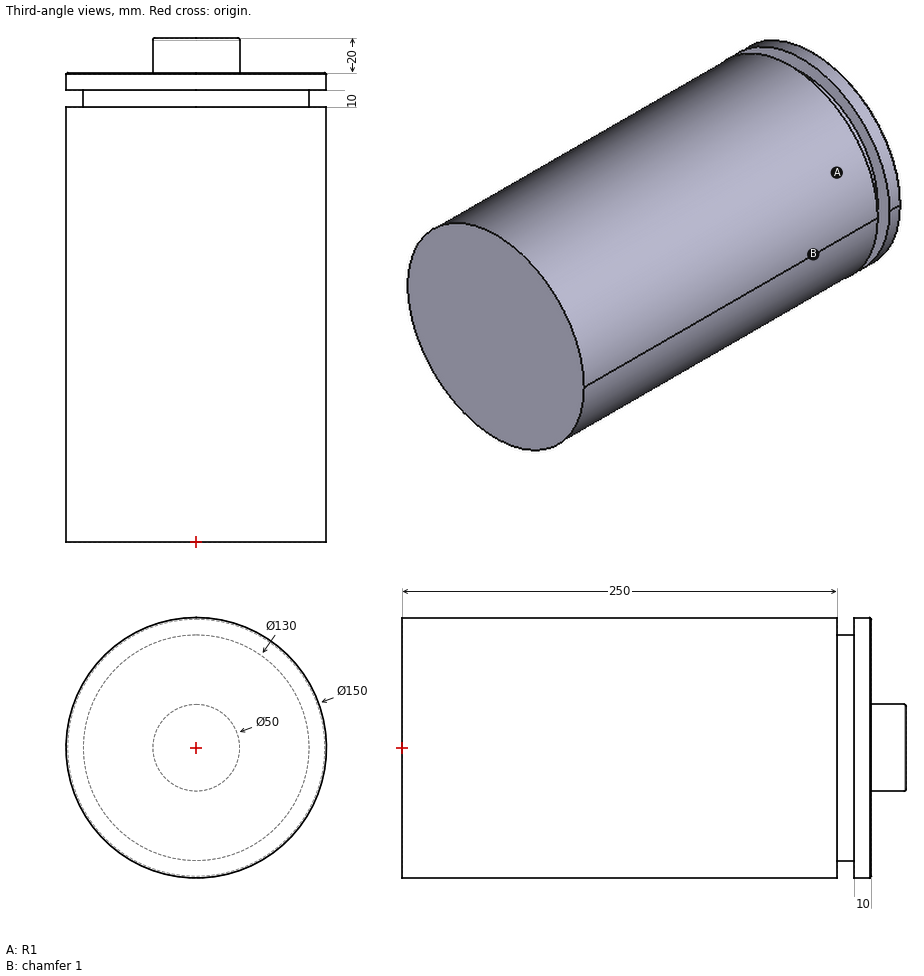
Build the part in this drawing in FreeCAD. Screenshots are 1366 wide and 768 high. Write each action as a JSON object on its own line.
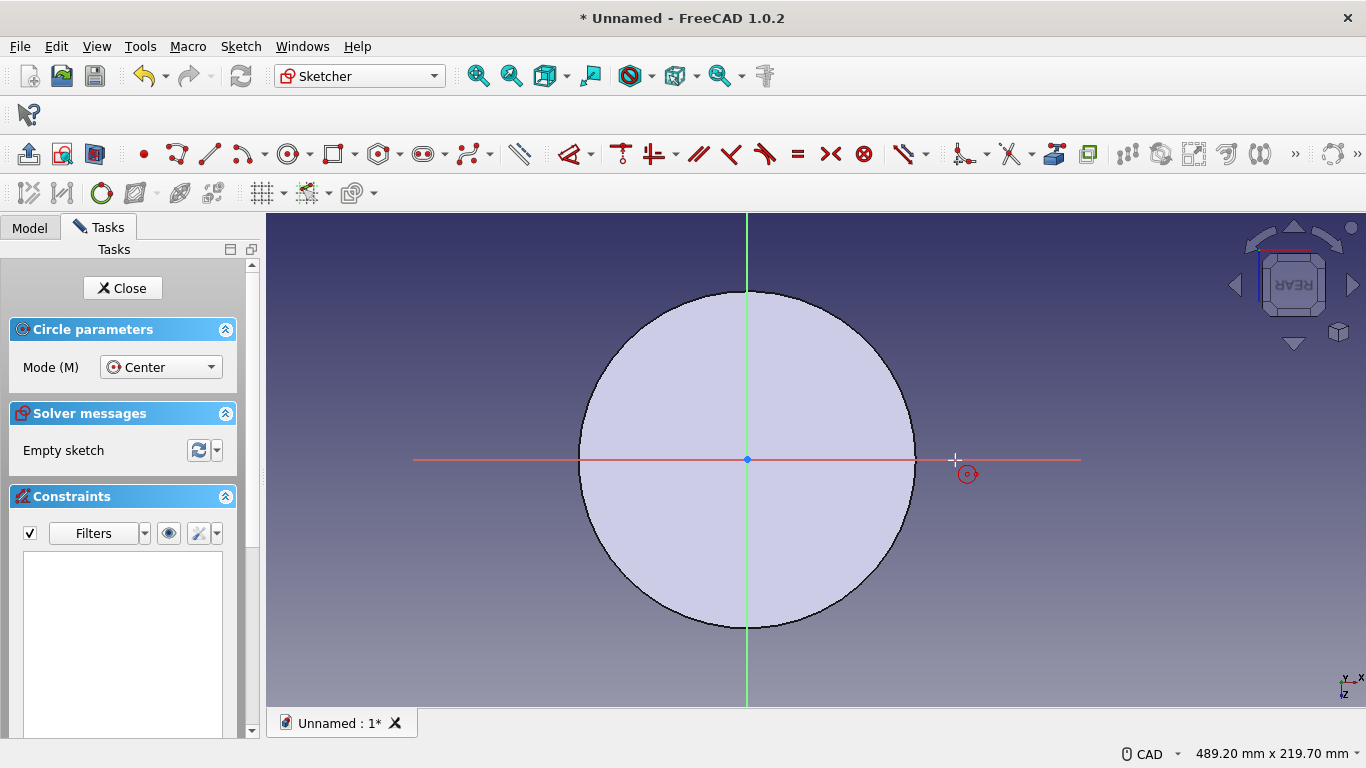
{"action": "left_click", "coordinate": [747, 460]}
{"action": "mouse_move", "coordinate": [850, 356]}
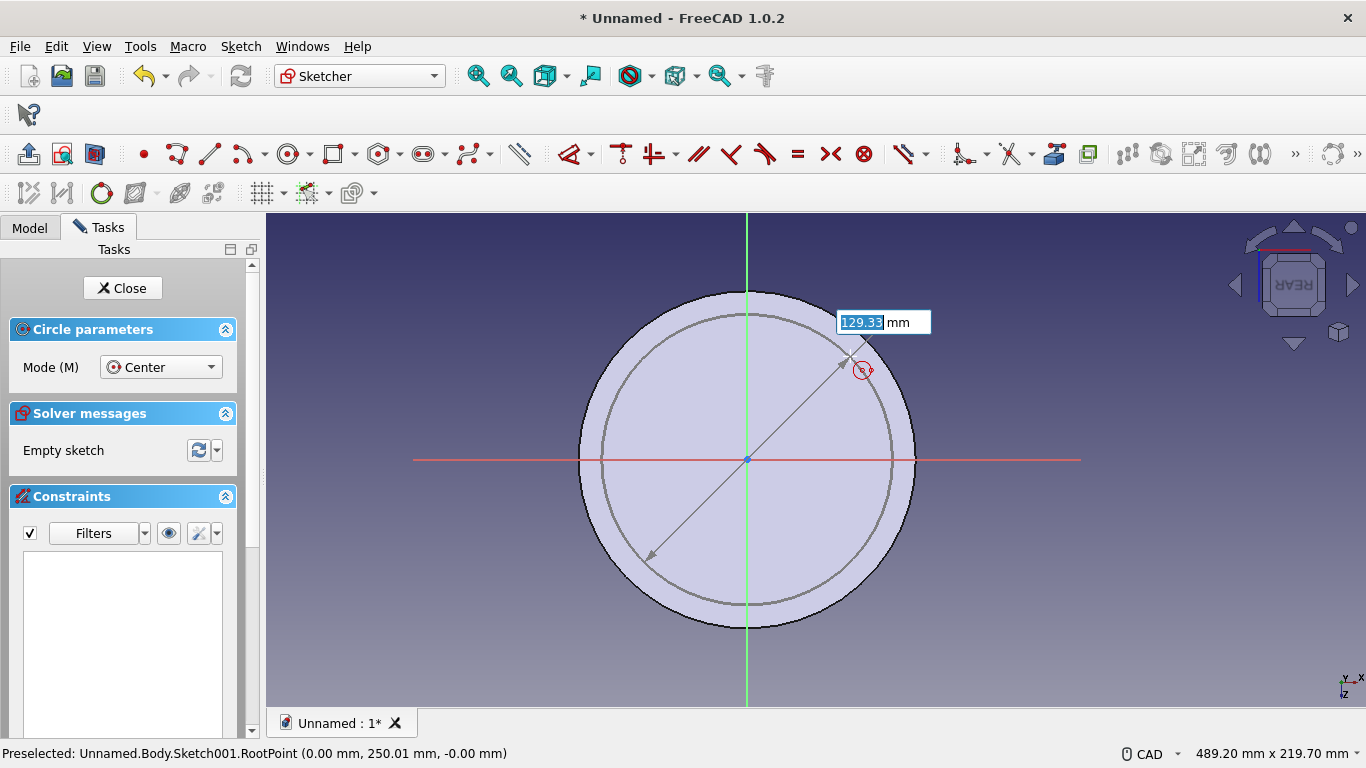
{"action": "type", "text": "130"}
{"action": "key", "text": "Return"}
{"action": "key", "text": "Escape"}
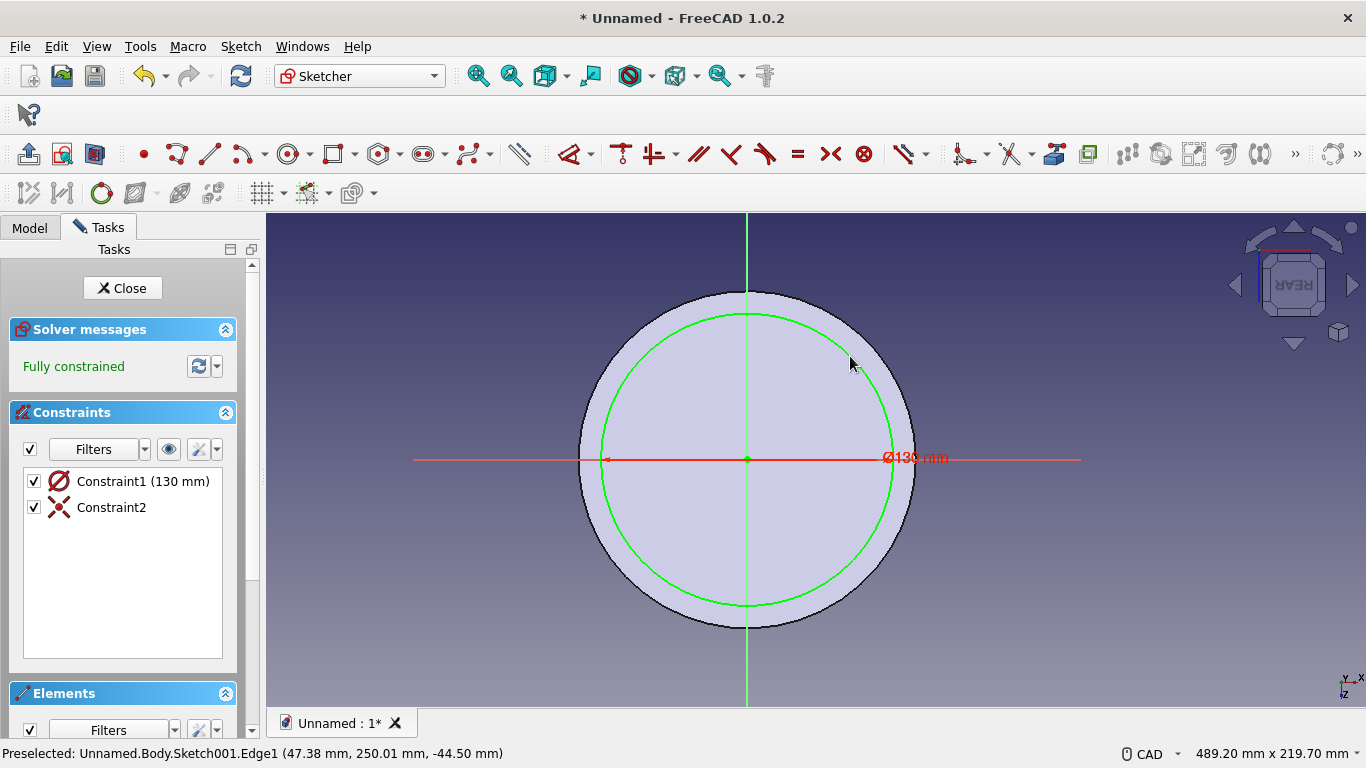
{"action": "left_click", "coordinate": [123, 288]}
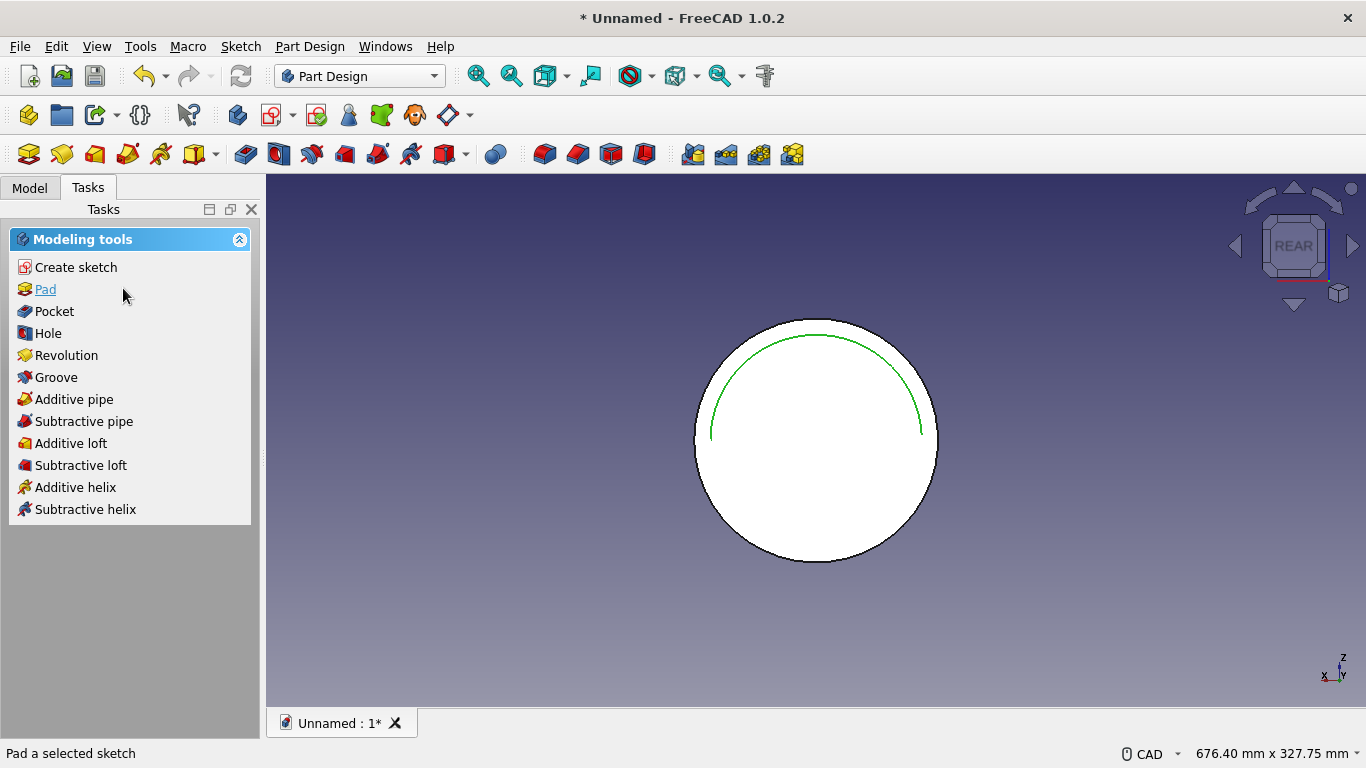
{"action": "left_click", "coordinate": [29, 154]}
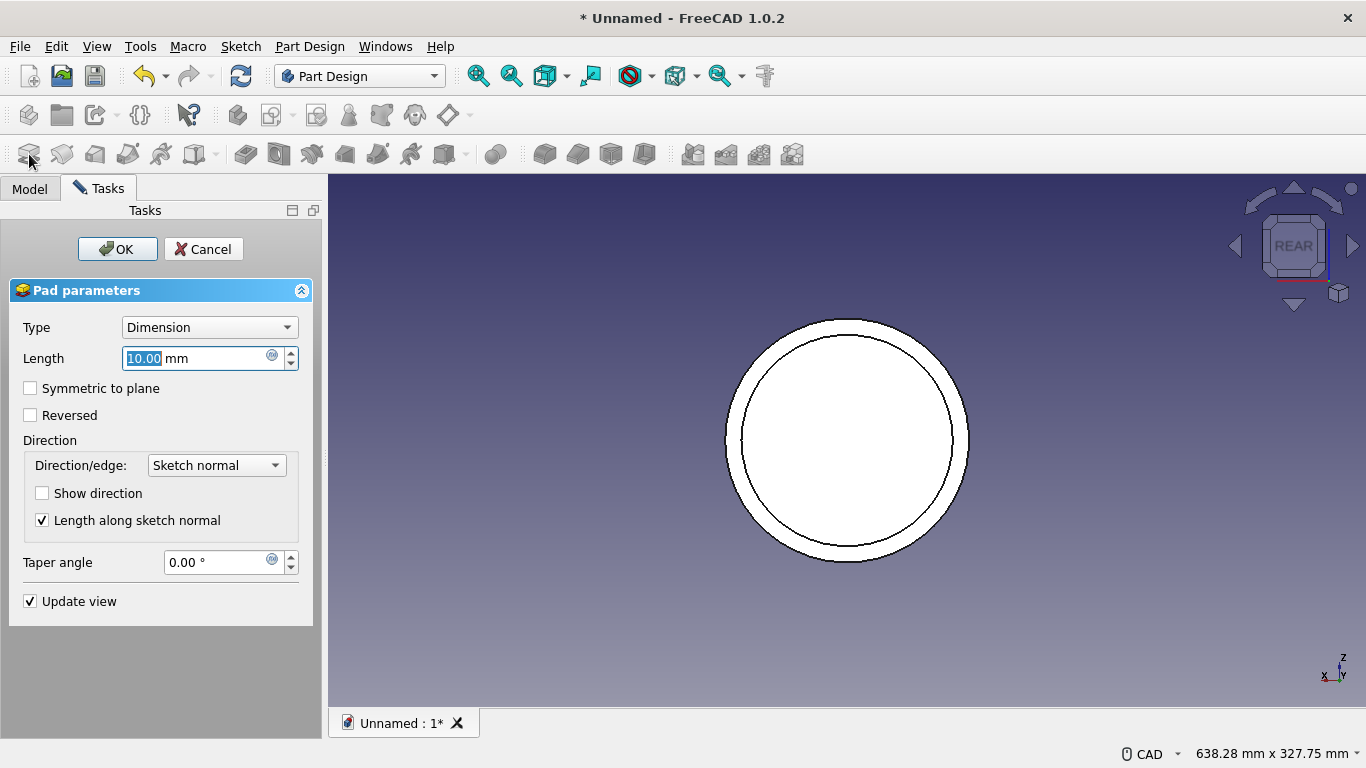
{"action": "type", "text": "10"}
{"action": "key", "text": "Tab"}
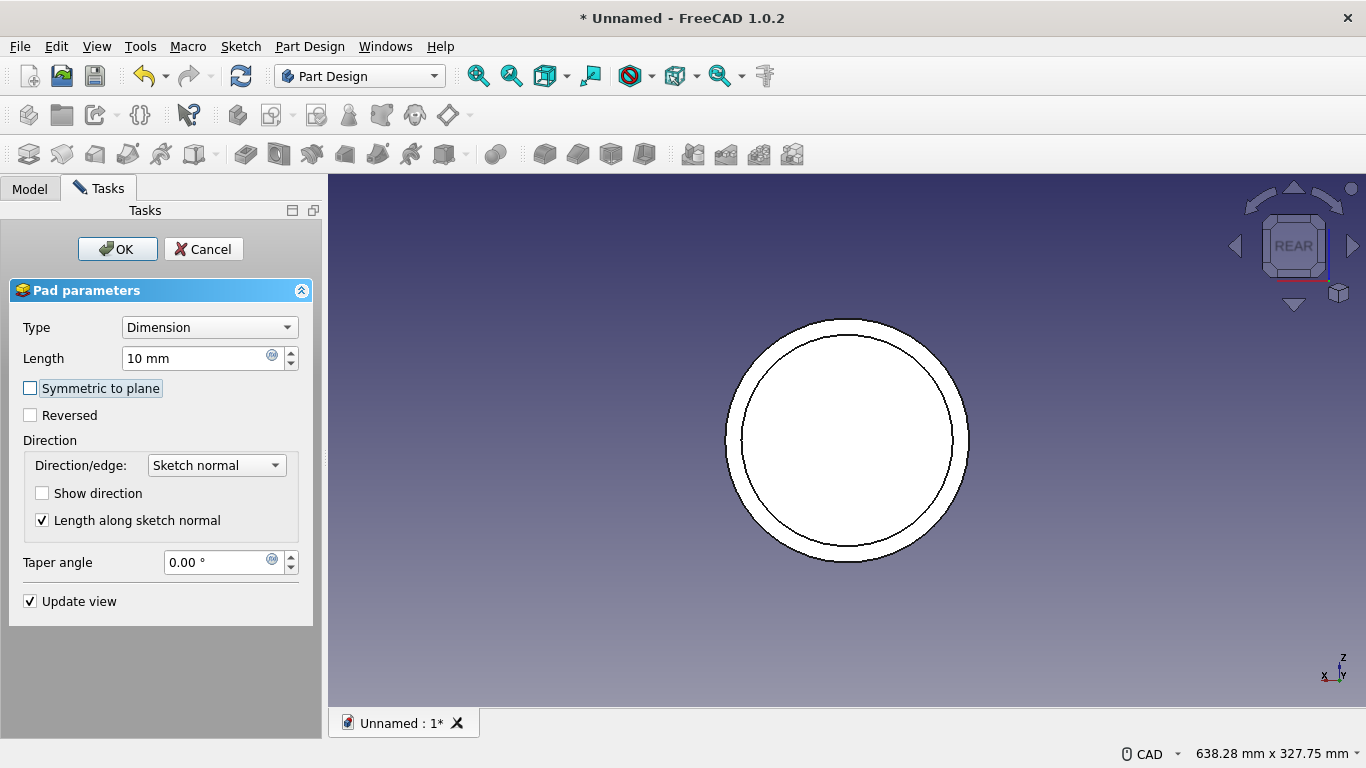
{"action": "left_click", "coordinate": [118, 249]}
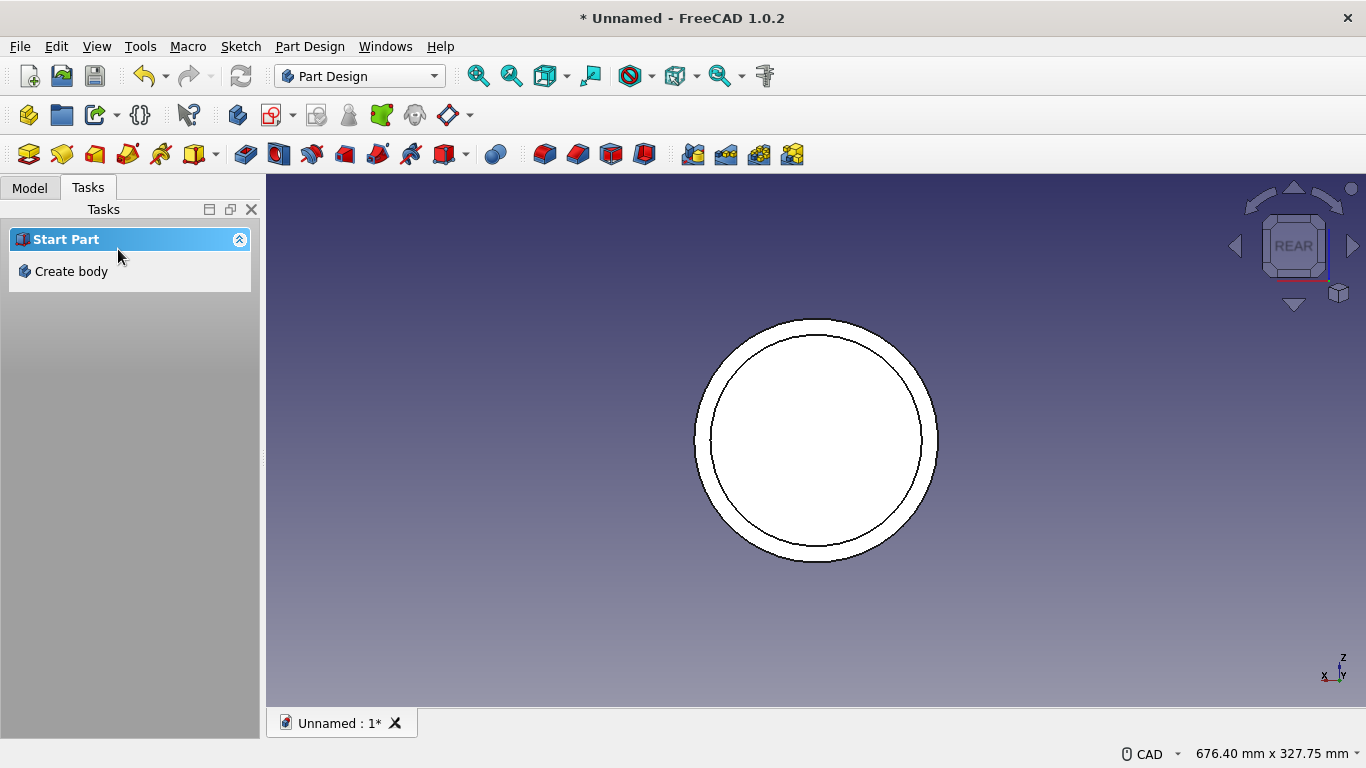
{"action": "left_click", "coordinate": [816, 440]}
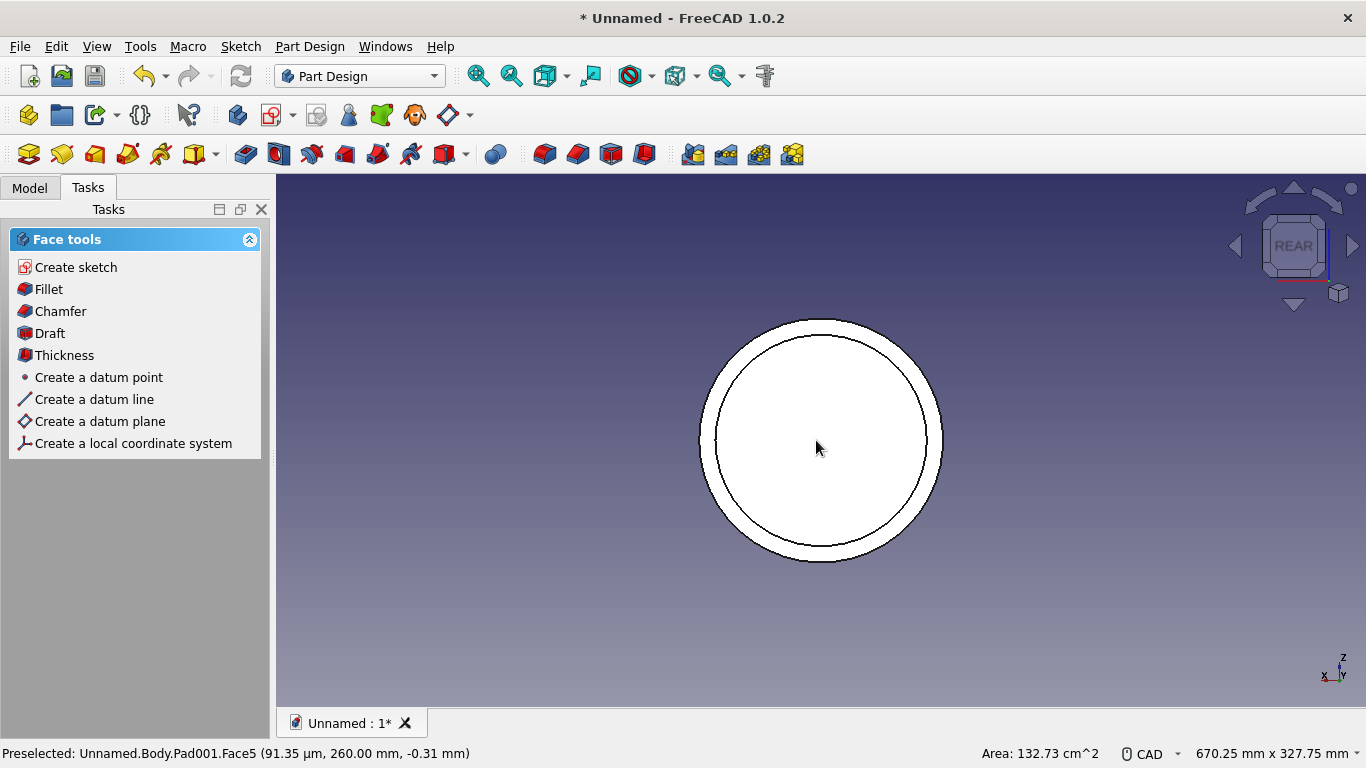
{"action": "left_click", "coordinate": [270, 116]}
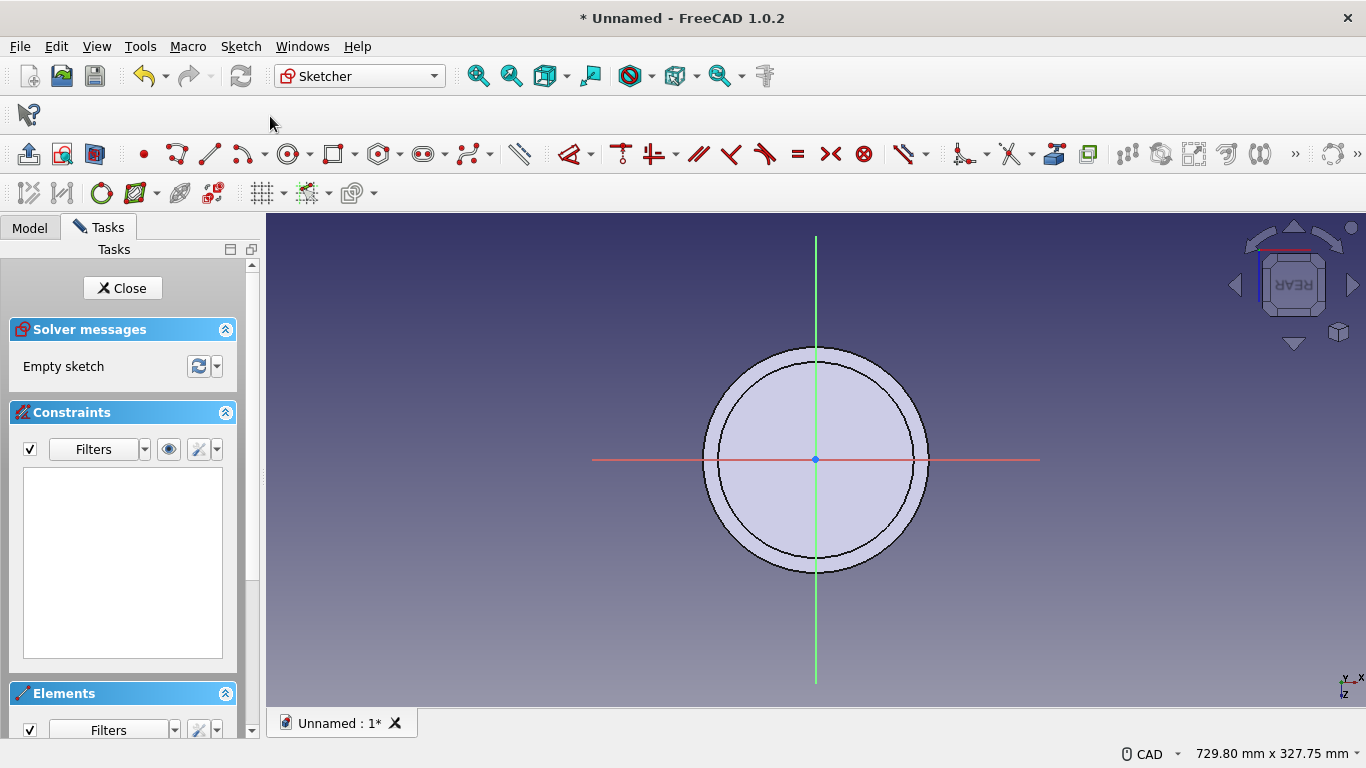
{"action": "scroll", "coordinate": [955, 460], "scroll_direction": "up", "scroll_amount": 2}